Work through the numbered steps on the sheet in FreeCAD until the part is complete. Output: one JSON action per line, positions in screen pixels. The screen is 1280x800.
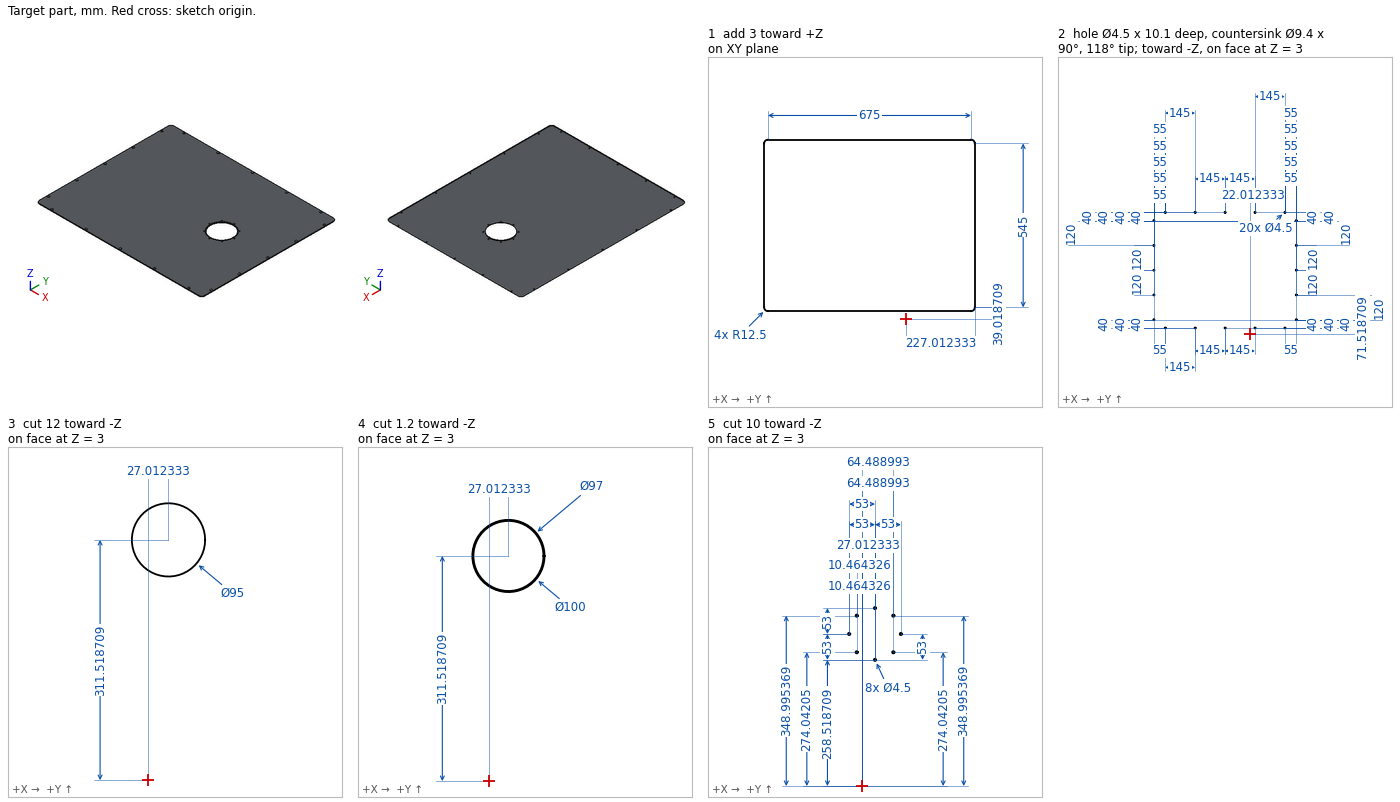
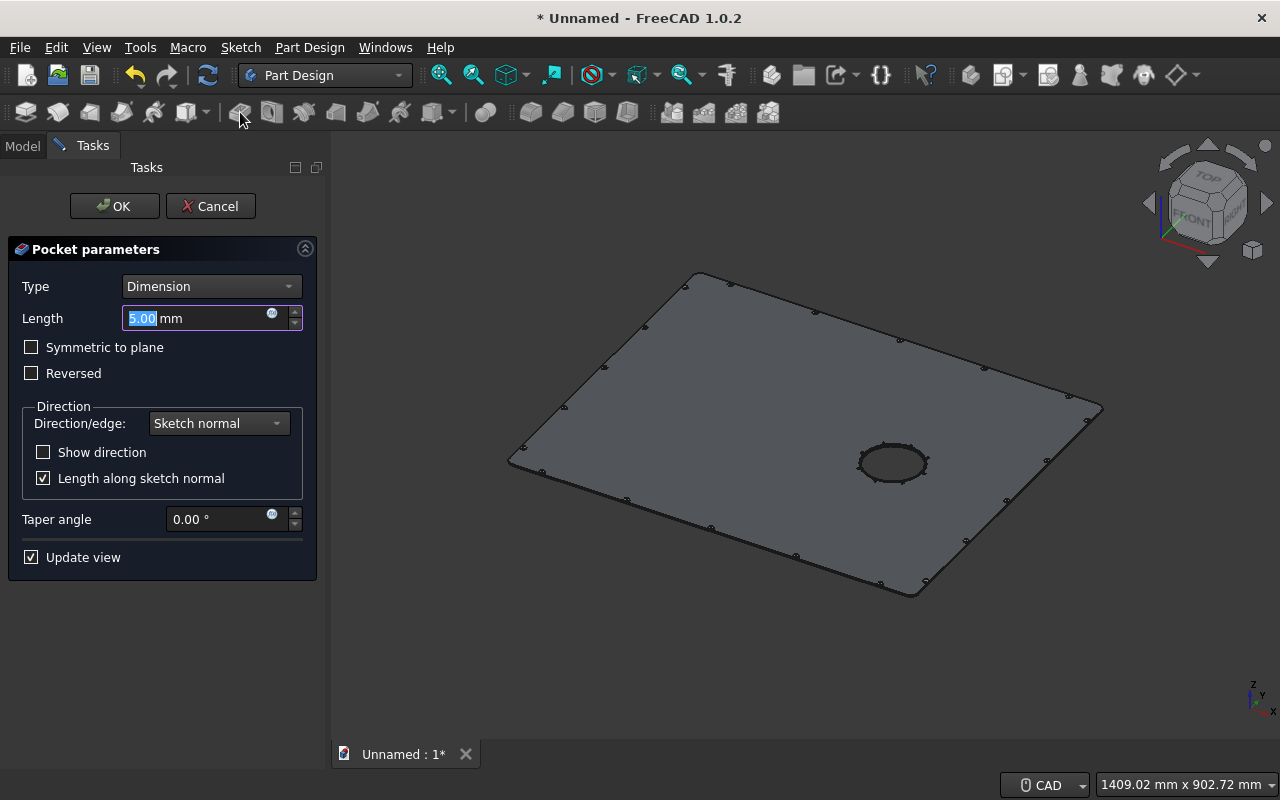
{"action": "type", "text": "10"}
{"action": "key", "text": "Tab"}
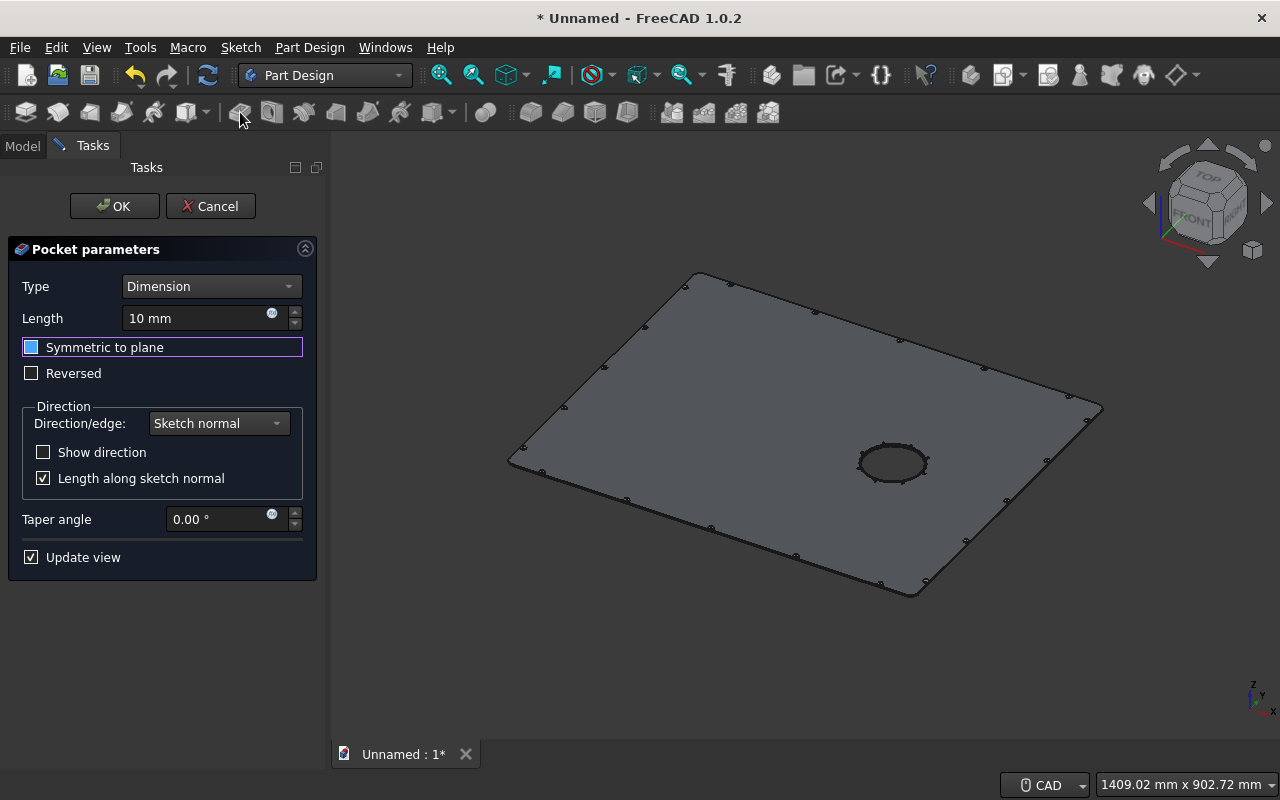
{"action": "left_click", "coordinate": [115, 206]}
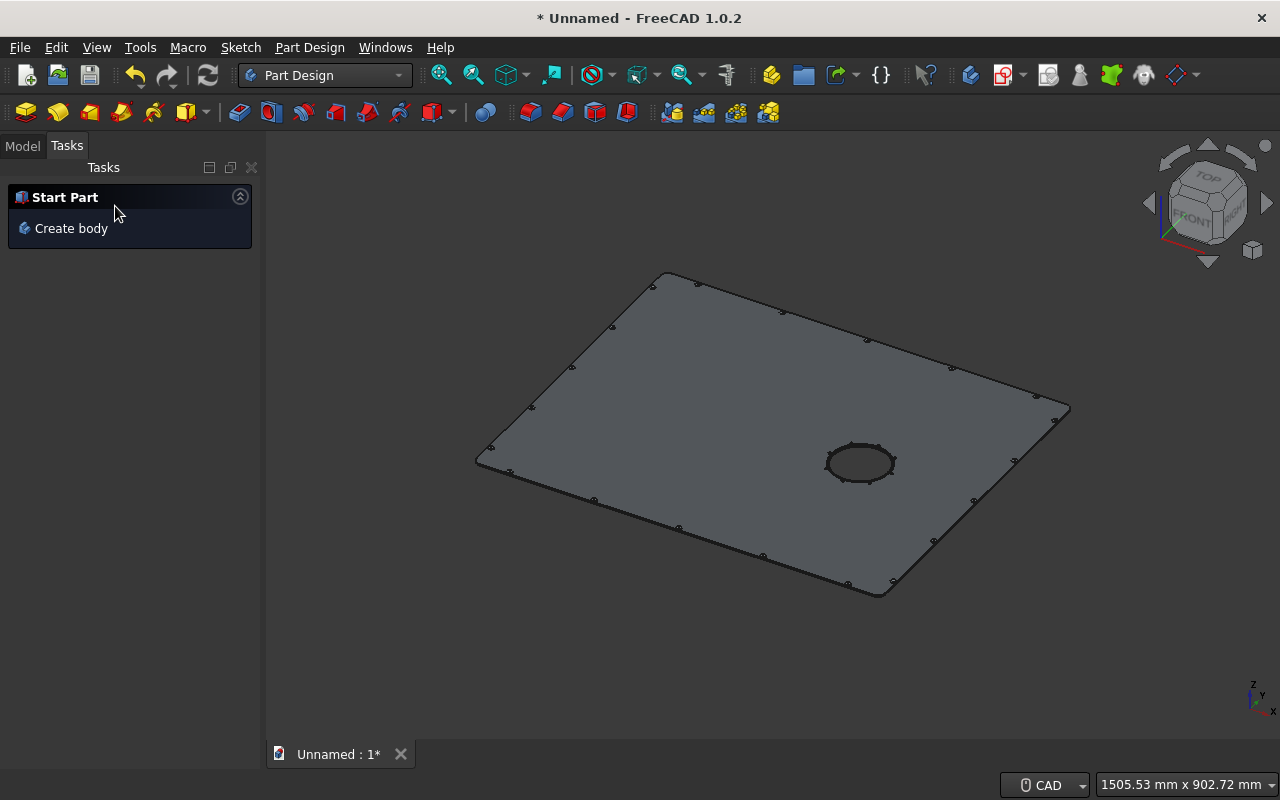
{"action": "key", "text": "0"}